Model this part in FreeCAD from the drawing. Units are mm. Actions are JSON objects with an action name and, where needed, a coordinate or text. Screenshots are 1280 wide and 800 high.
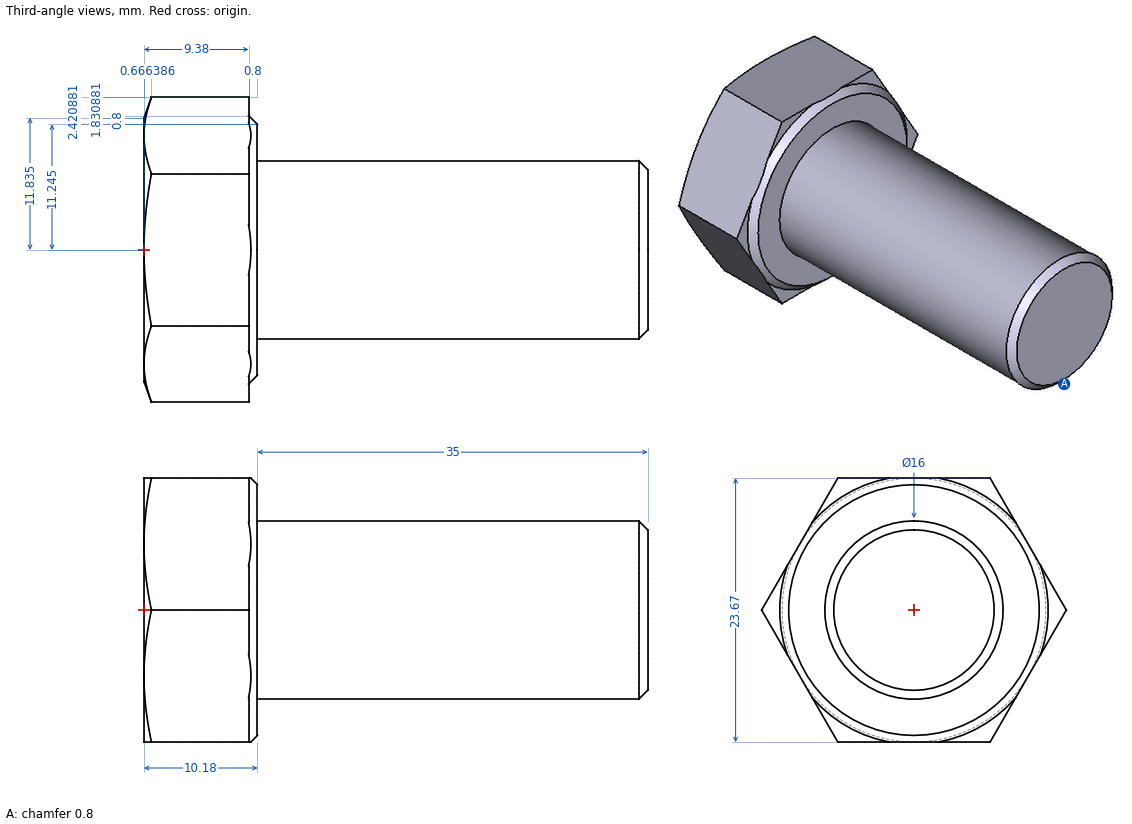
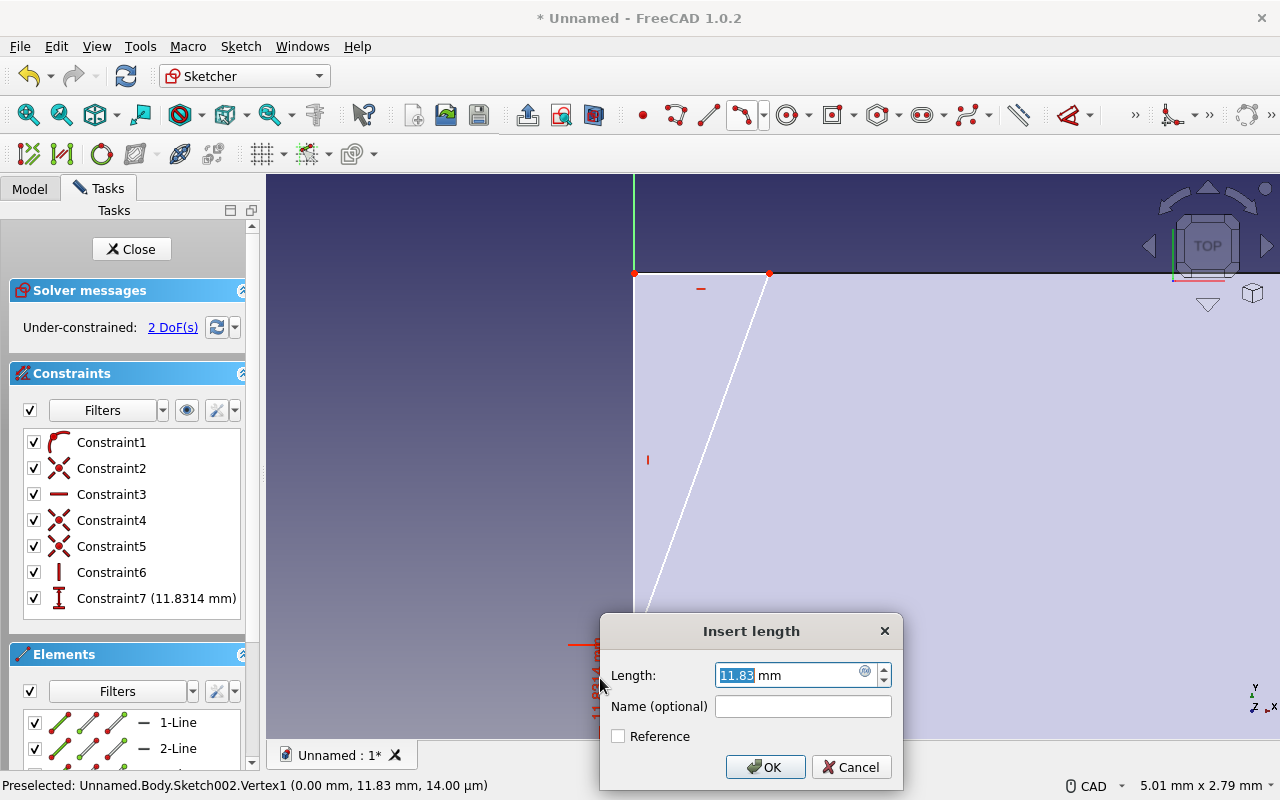
{"action": "type", "text": "11.835"}
{"action": "key", "text": "Return"}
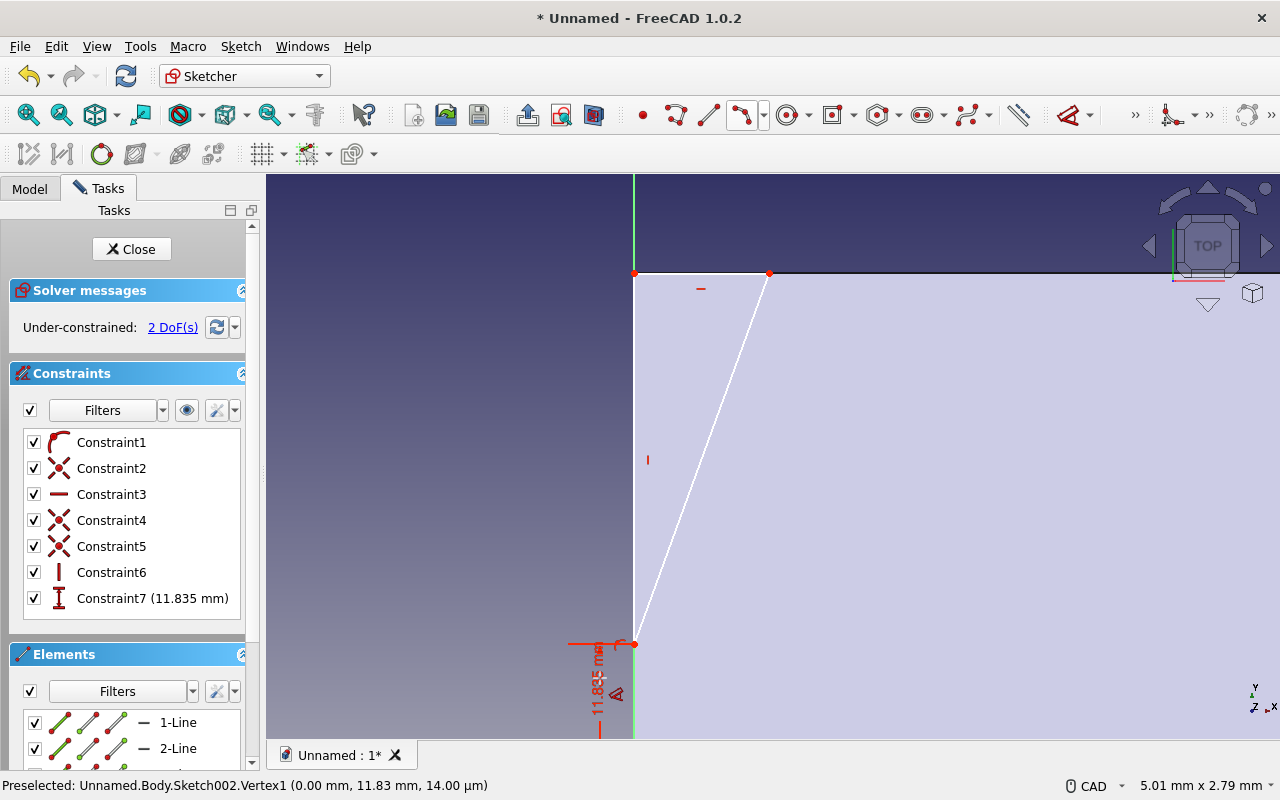
{"action": "left_click", "coordinate": [729, 274]}
{"action": "left_click", "coordinate": [702, 240]}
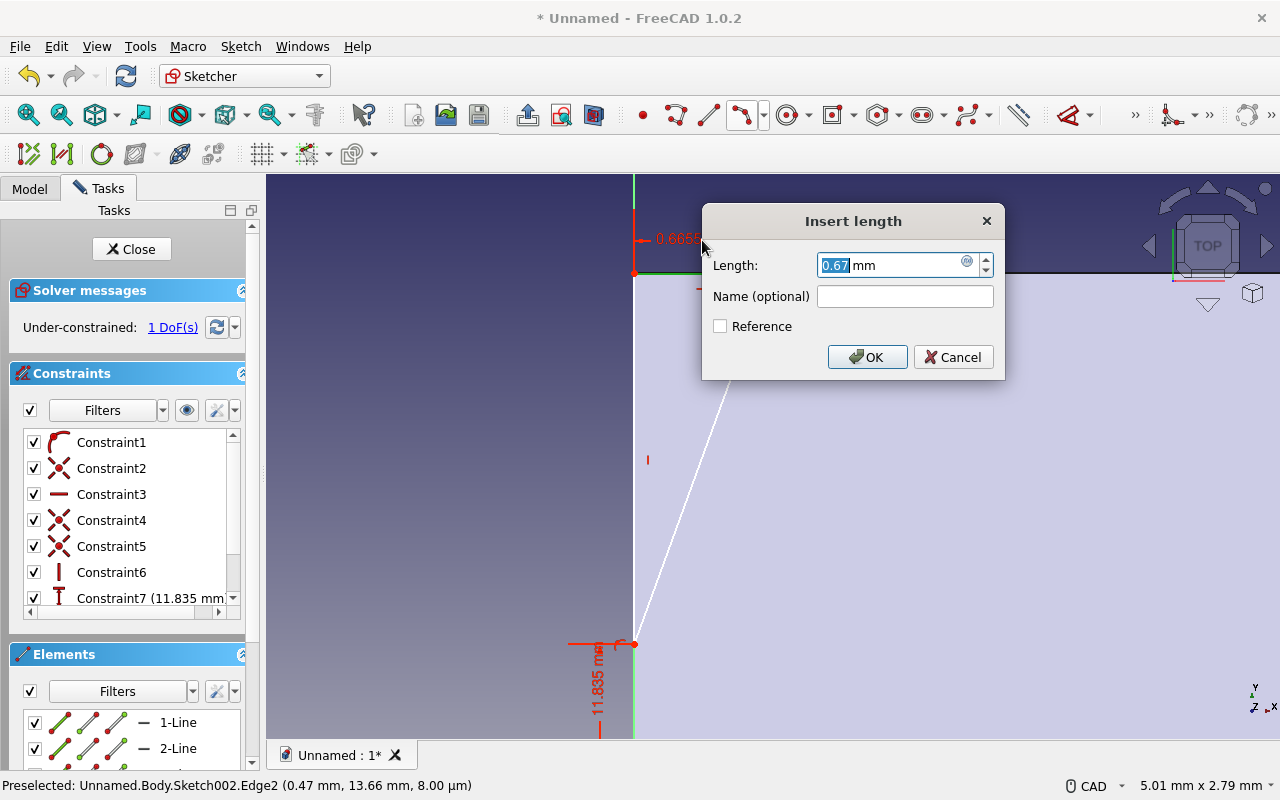
{"action": "type", "text": "0.666386"}
{"action": "key", "text": "Return"}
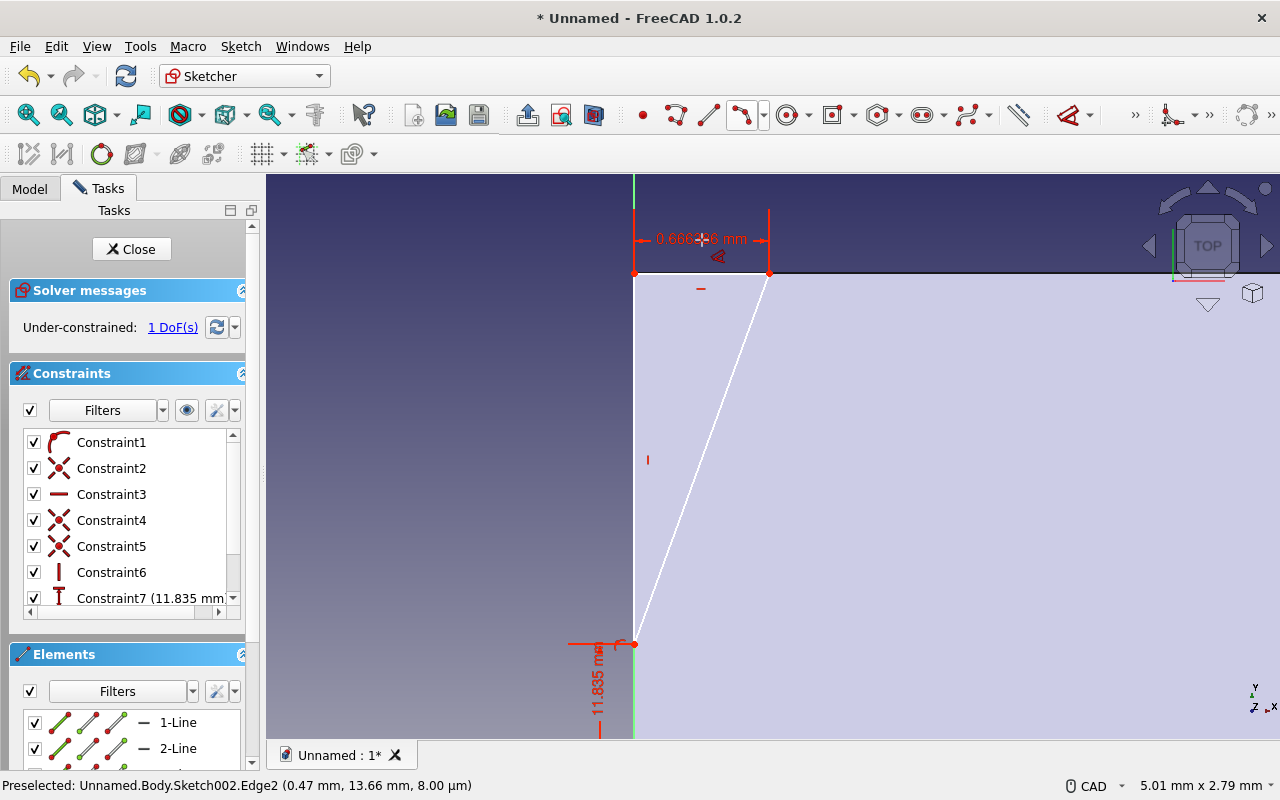
{"action": "left_click", "coordinate": [634, 385]}
{"action": "left_click", "coordinate": [600, 459]}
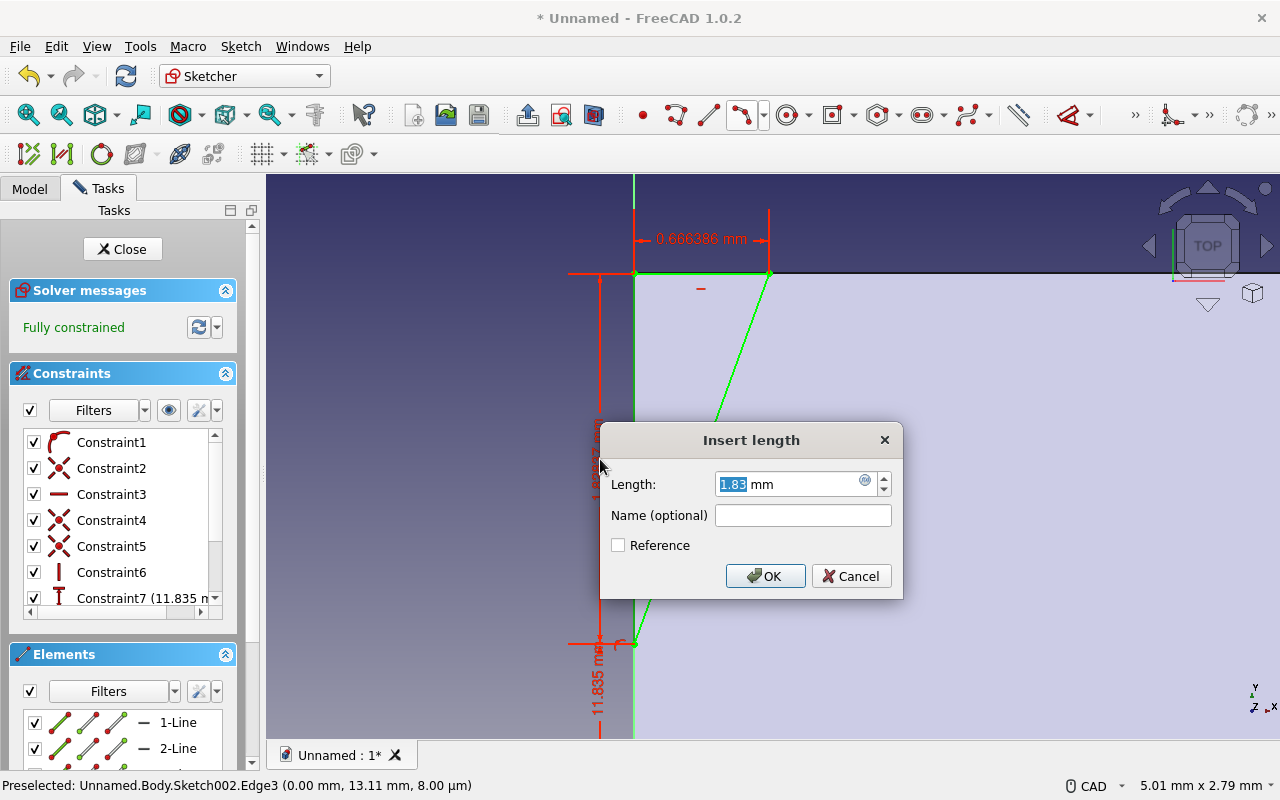
{"action": "type", "text": "1.830881"}
{"action": "key", "text": "Return"}
{"action": "key", "text": "Escape"}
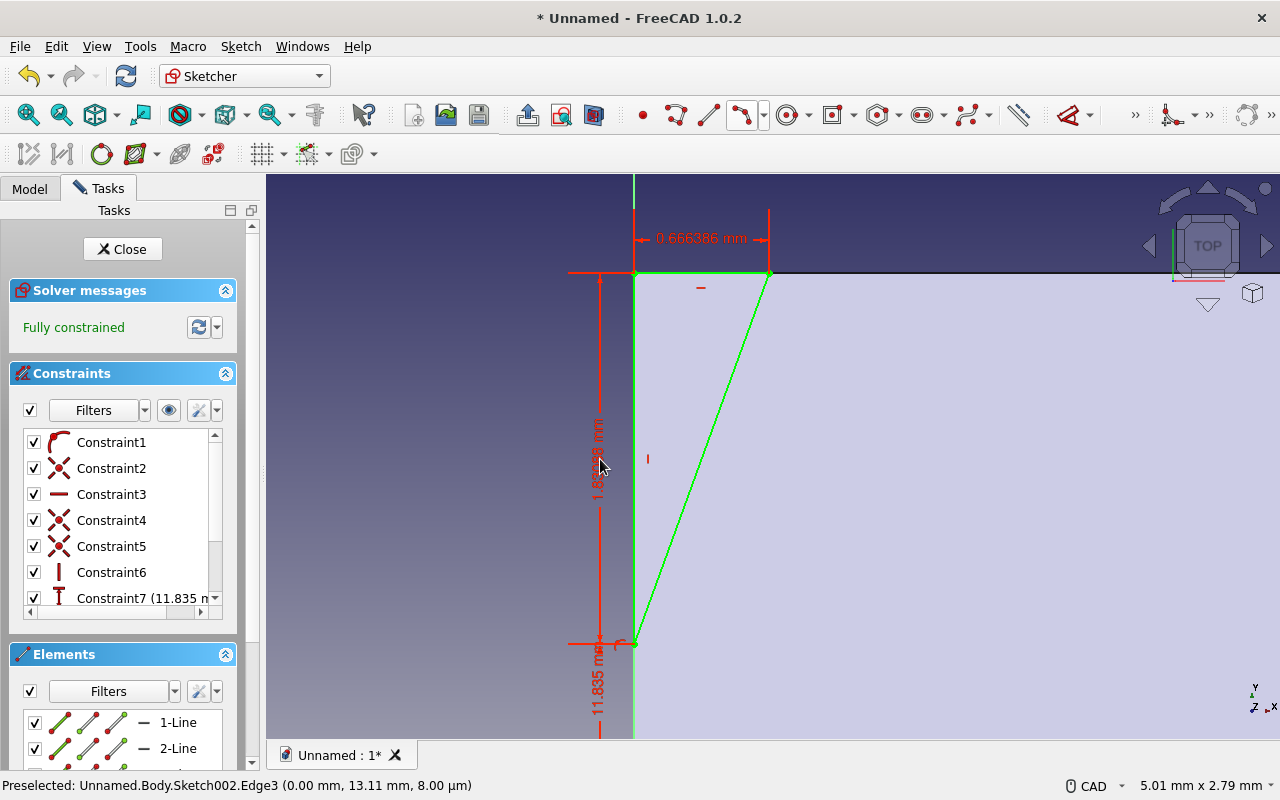
{"action": "left_click", "coordinate": [123, 249]}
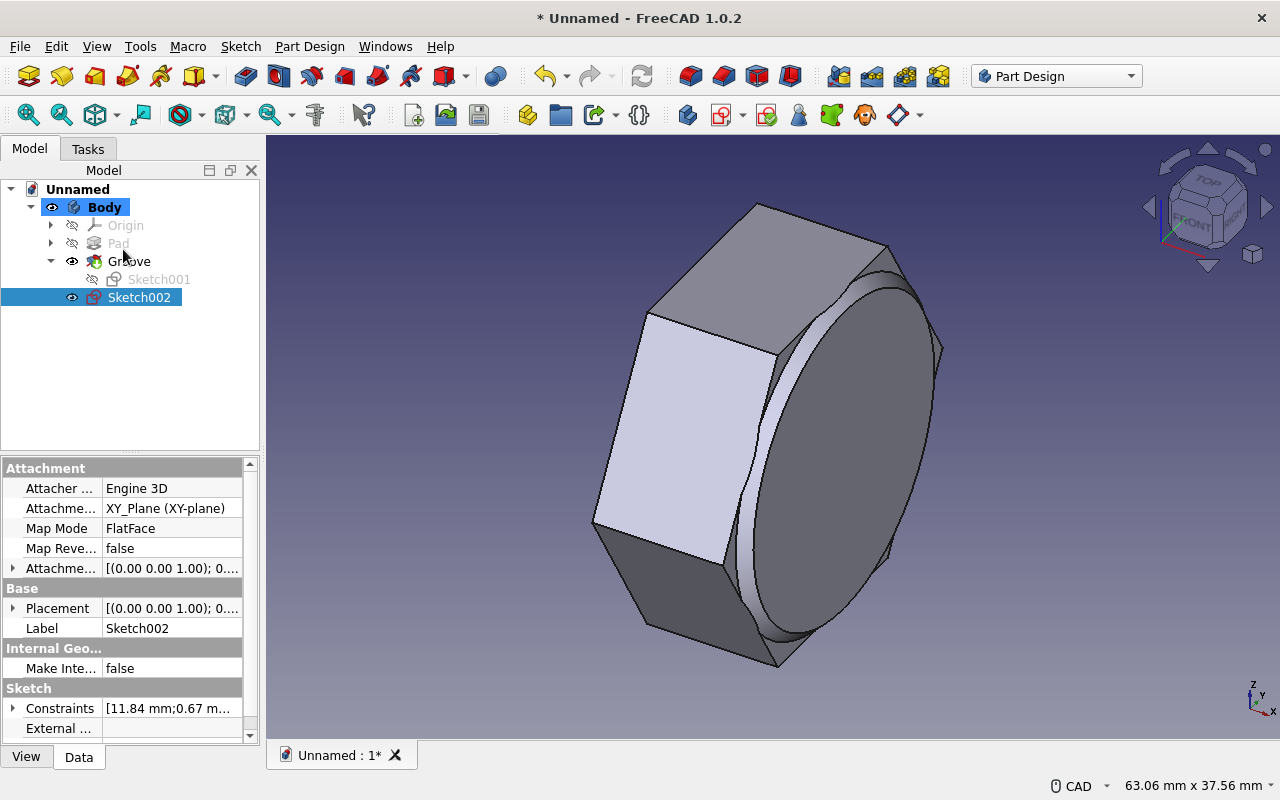
{"action": "left_click", "coordinate": [312, 76]}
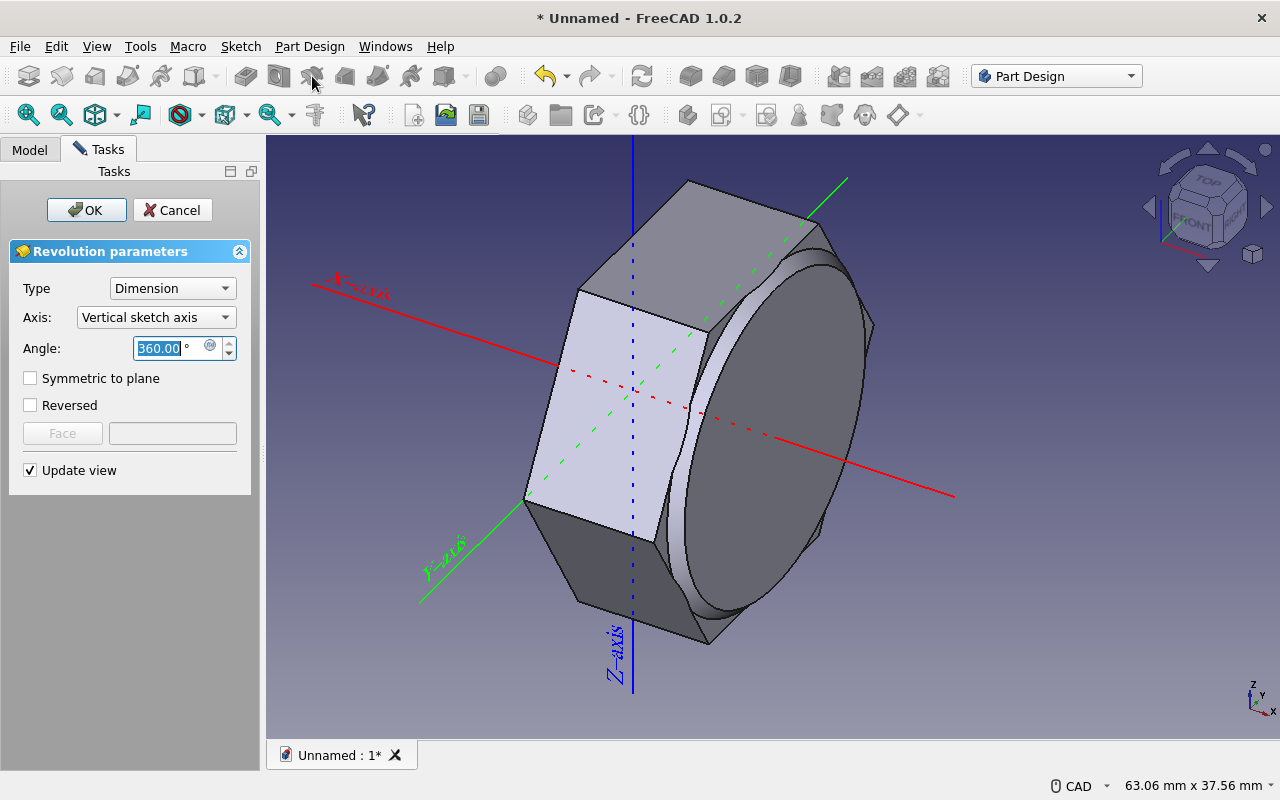
{"action": "left_click", "coordinate": [157, 318]}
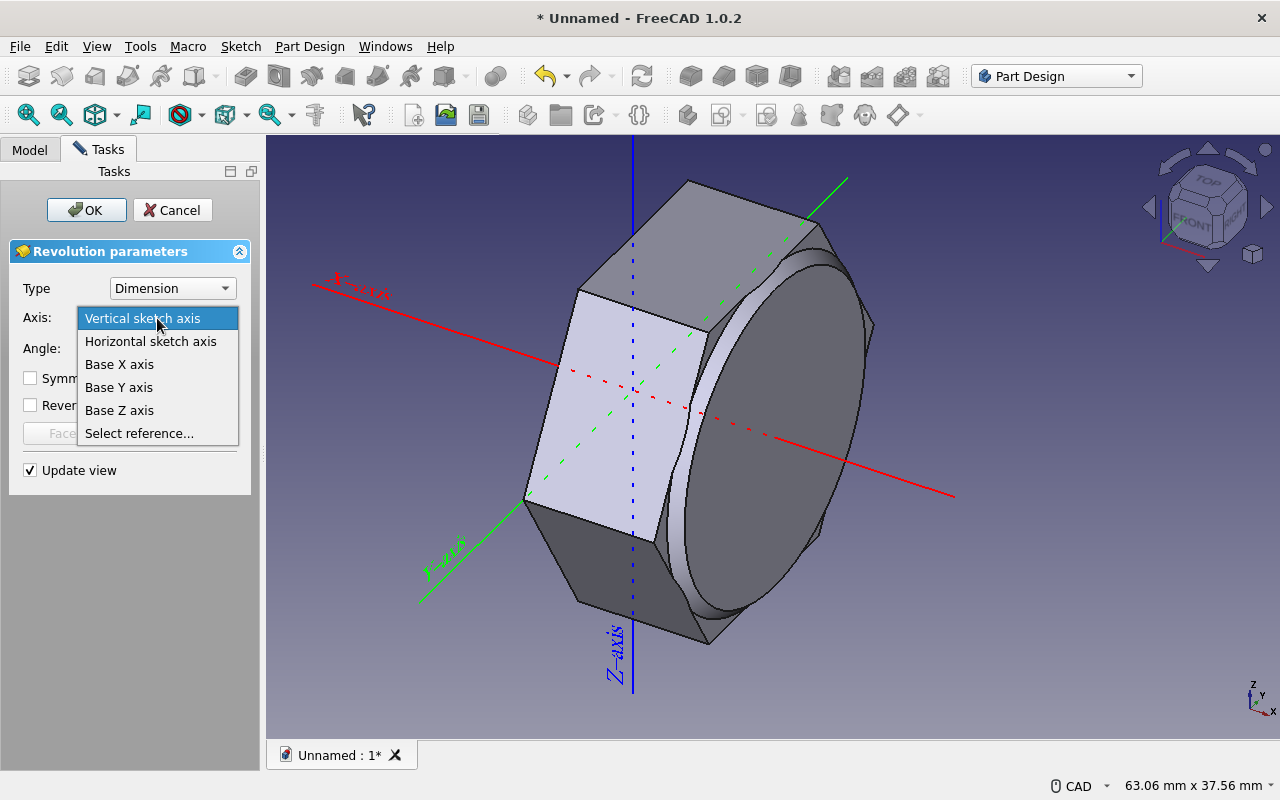
{"action": "left_click", "coordinate": [156, 342]}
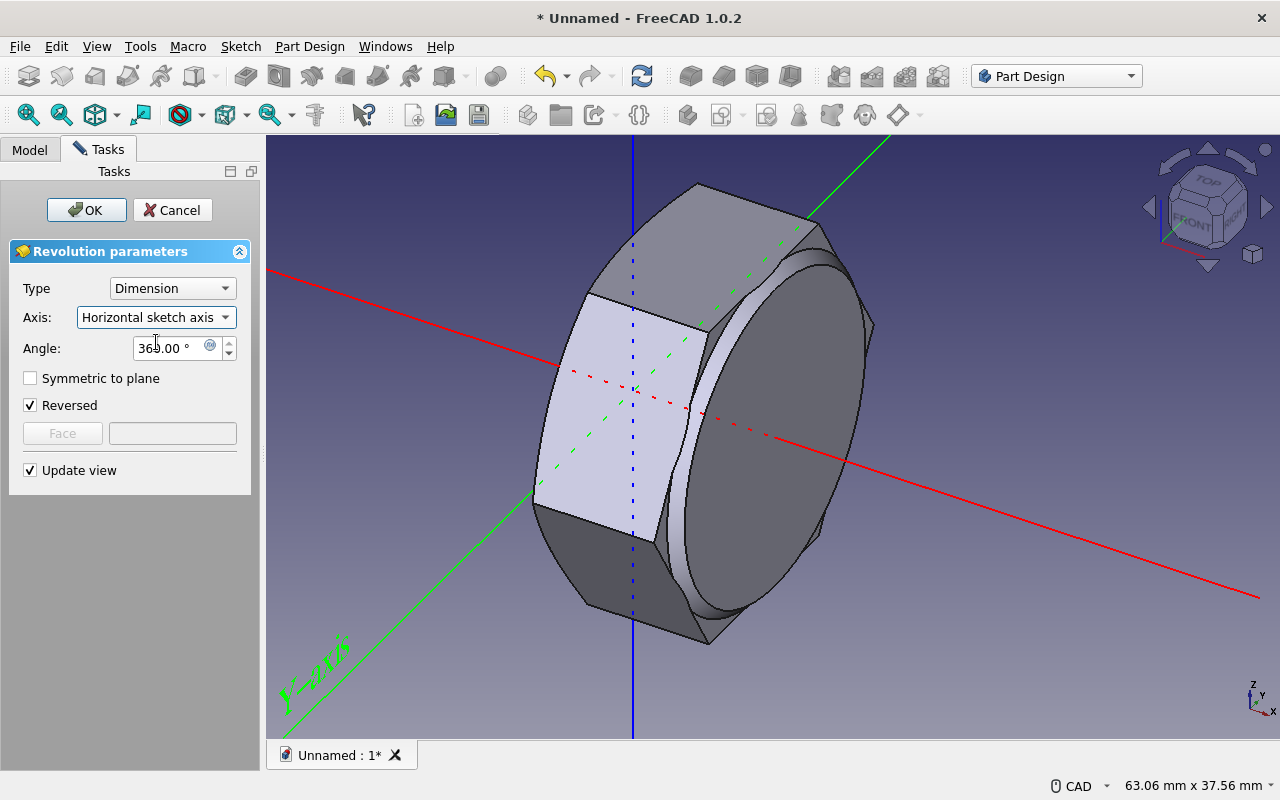
{"action": "left_click", "coordinate": [87, 210]}